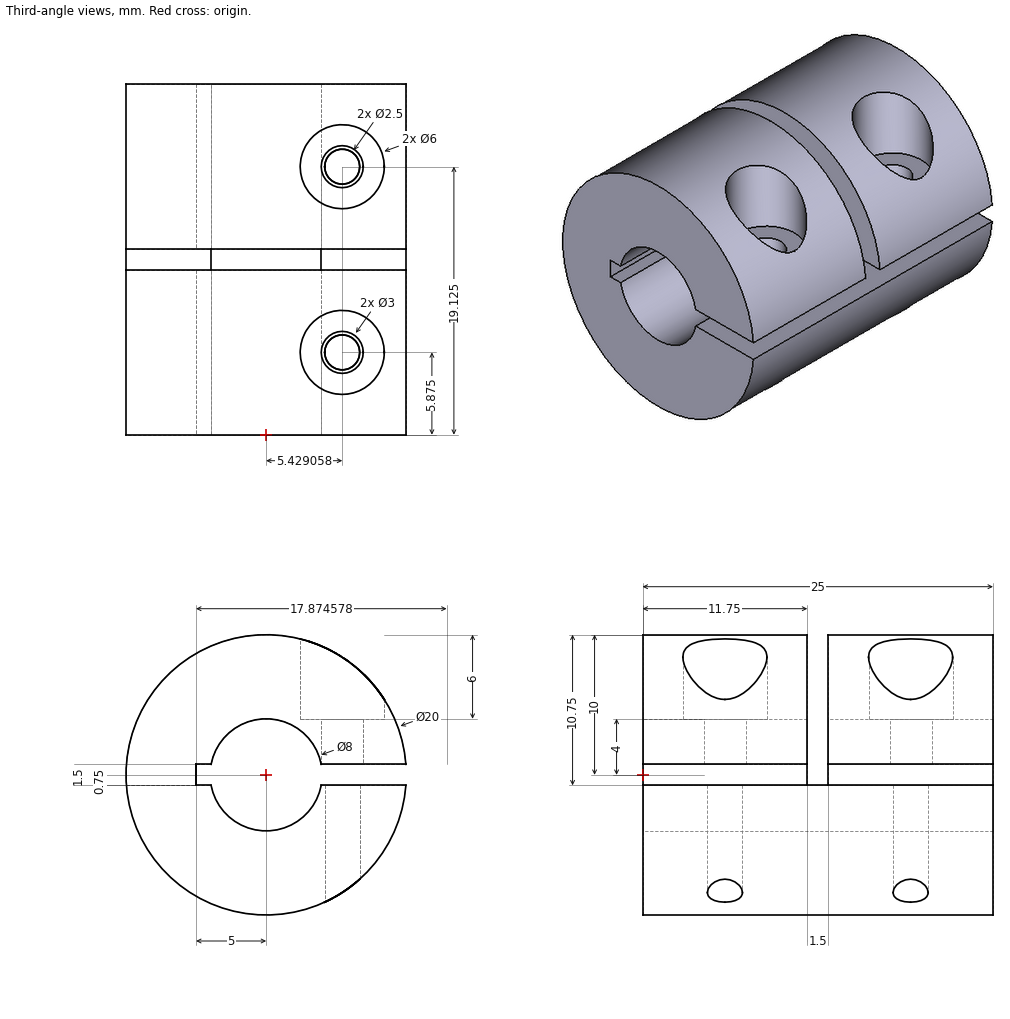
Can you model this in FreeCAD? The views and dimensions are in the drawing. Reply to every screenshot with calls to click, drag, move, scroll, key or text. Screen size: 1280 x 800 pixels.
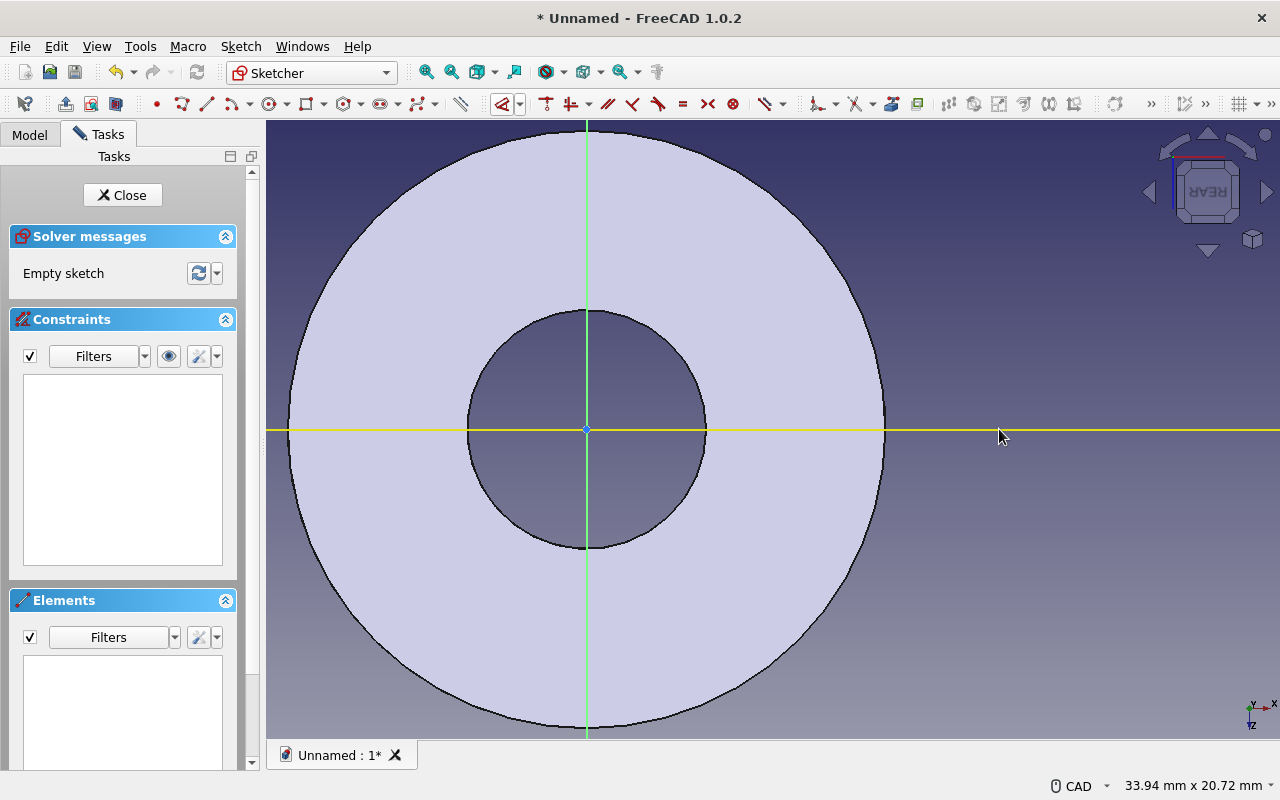
click(306, 104)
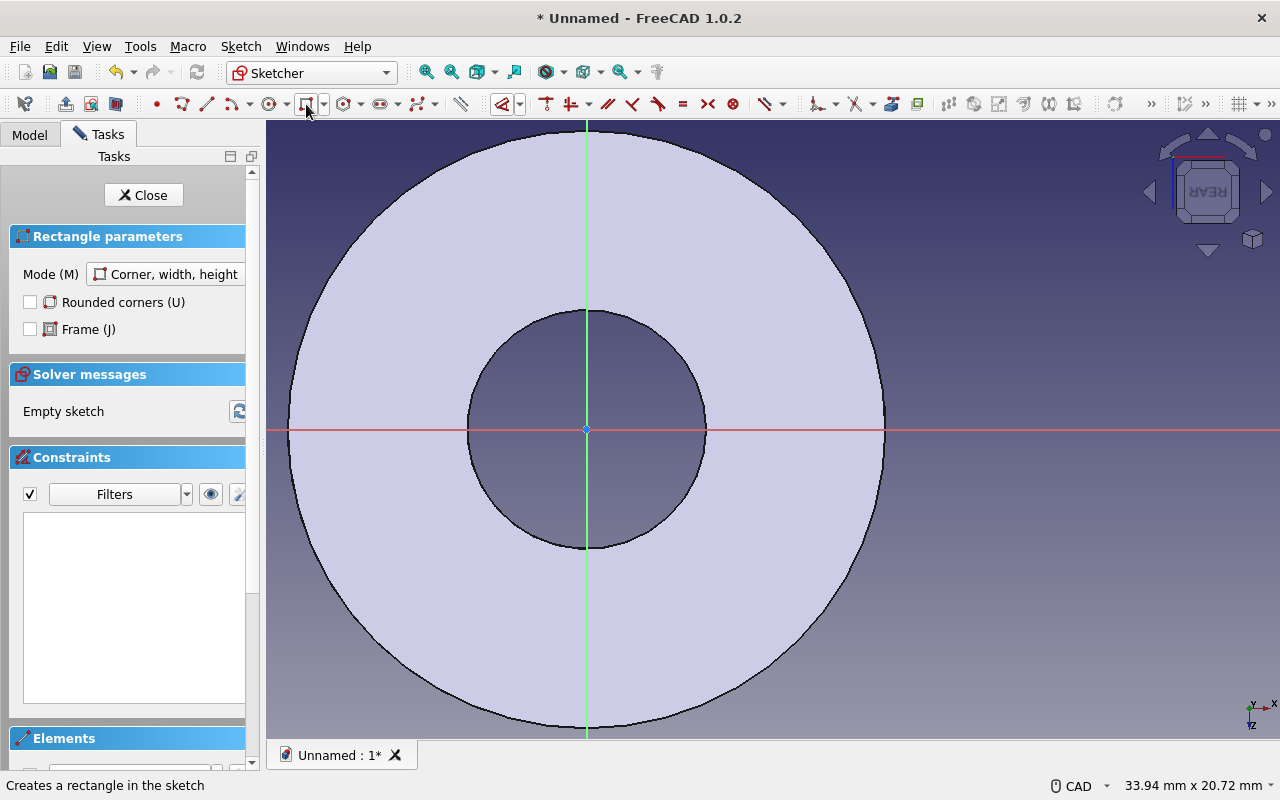
click(437, 407)
click(971, 452)
key(Escape)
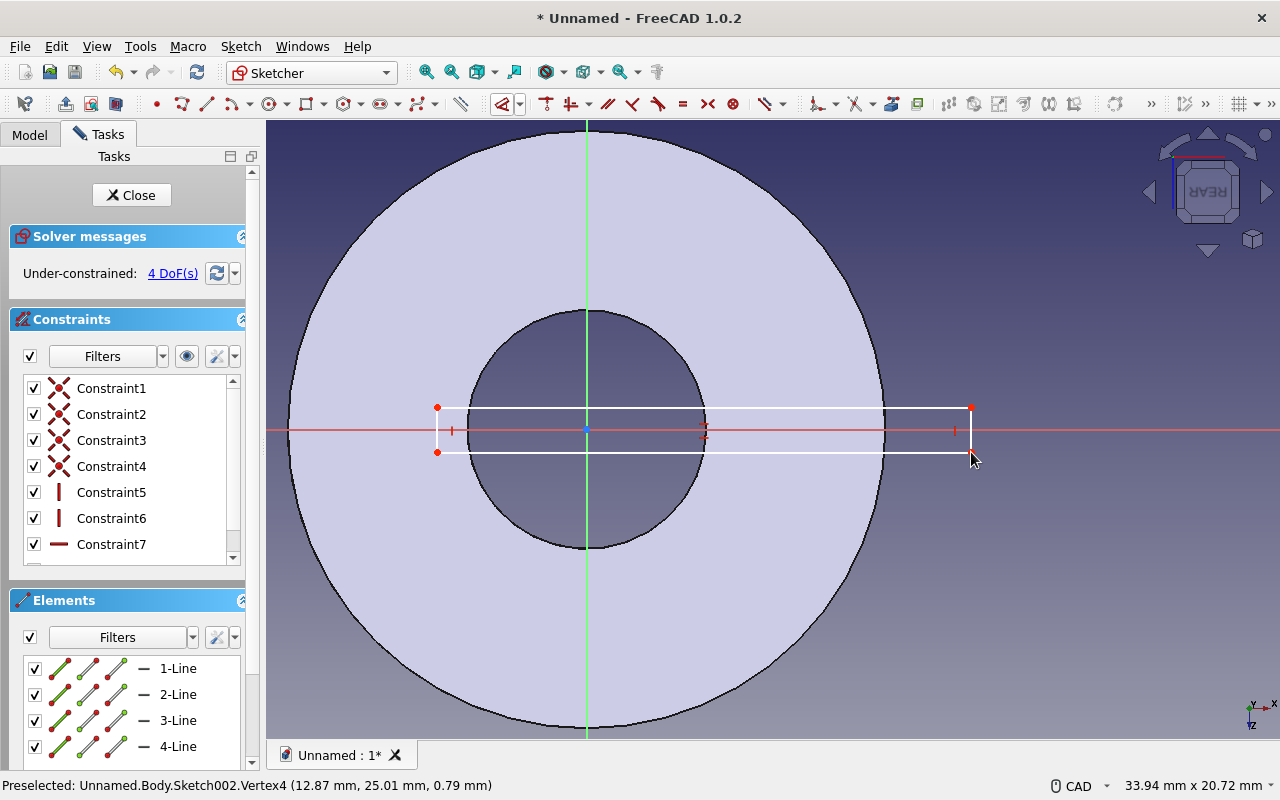
click(437, 408)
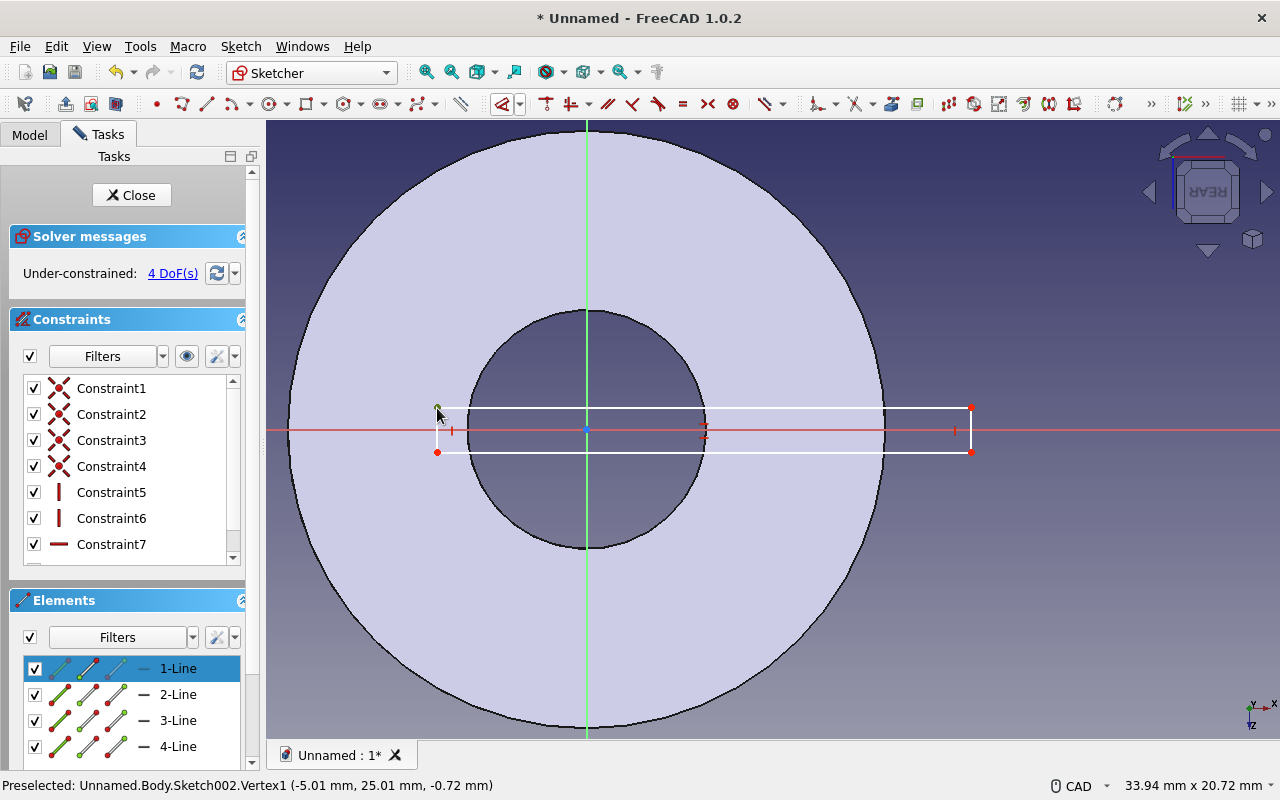
click(520, 104)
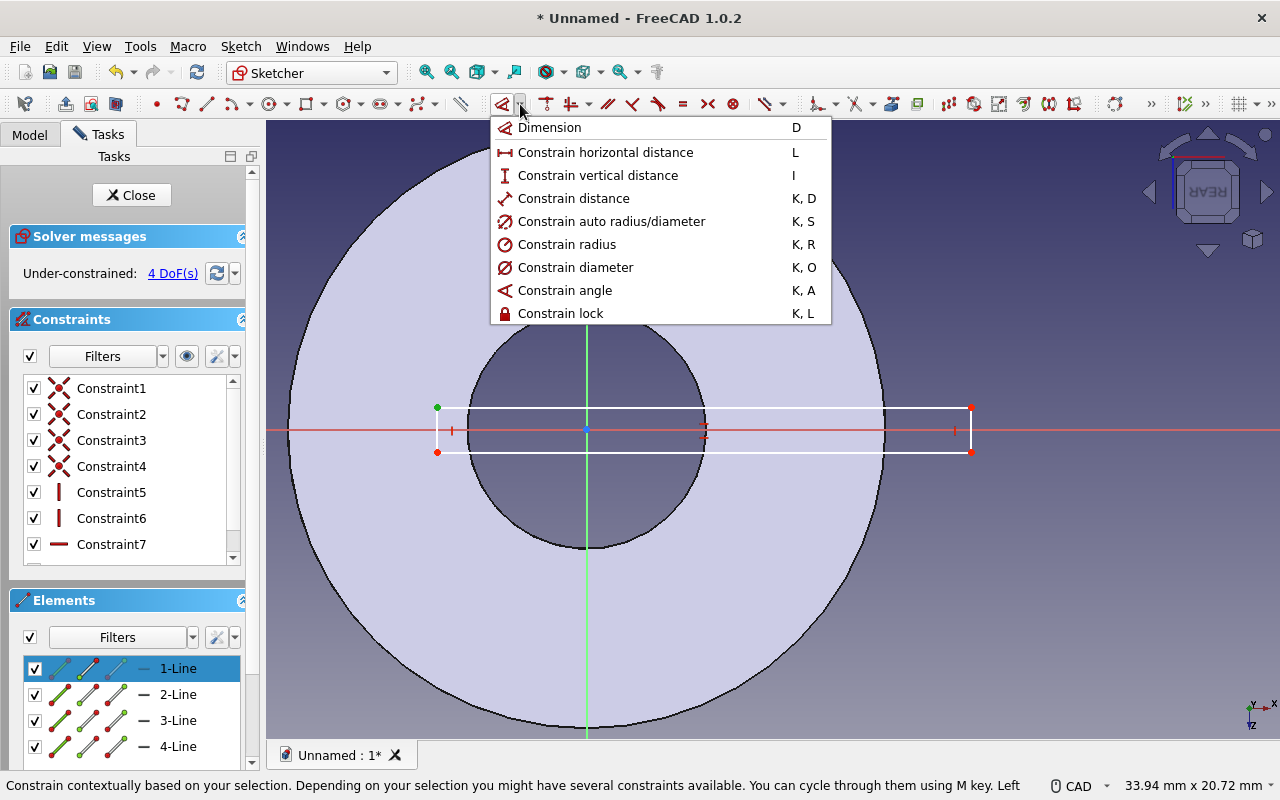
click(661, 152)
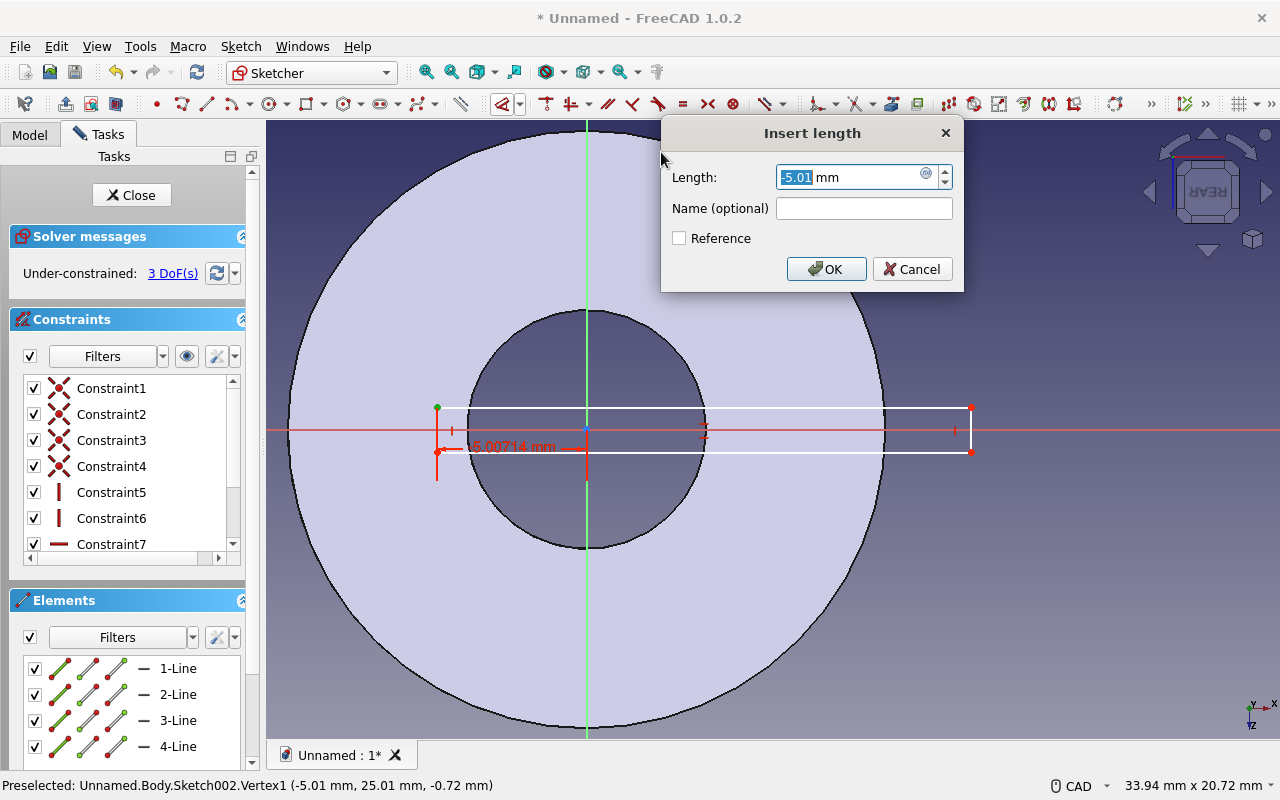
text(-5)
key(Return)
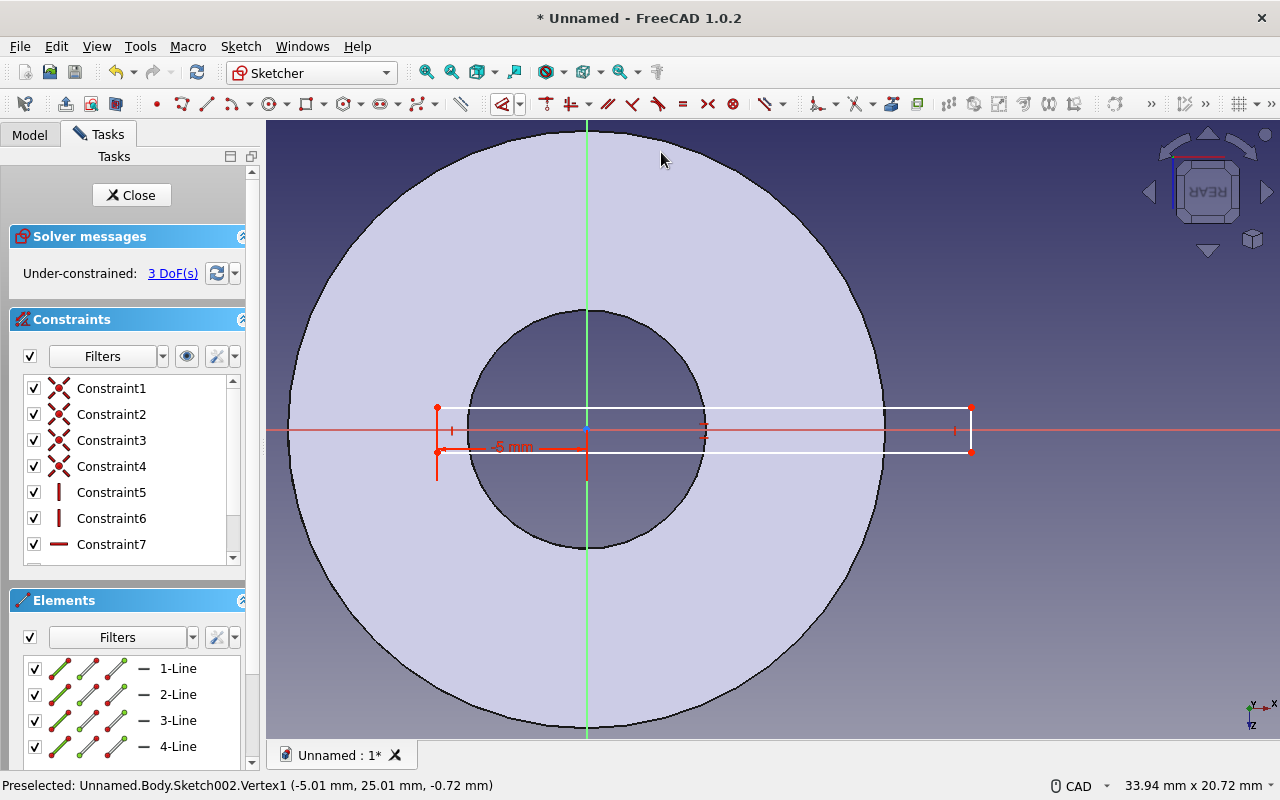
scroll(437, 440, up, 2)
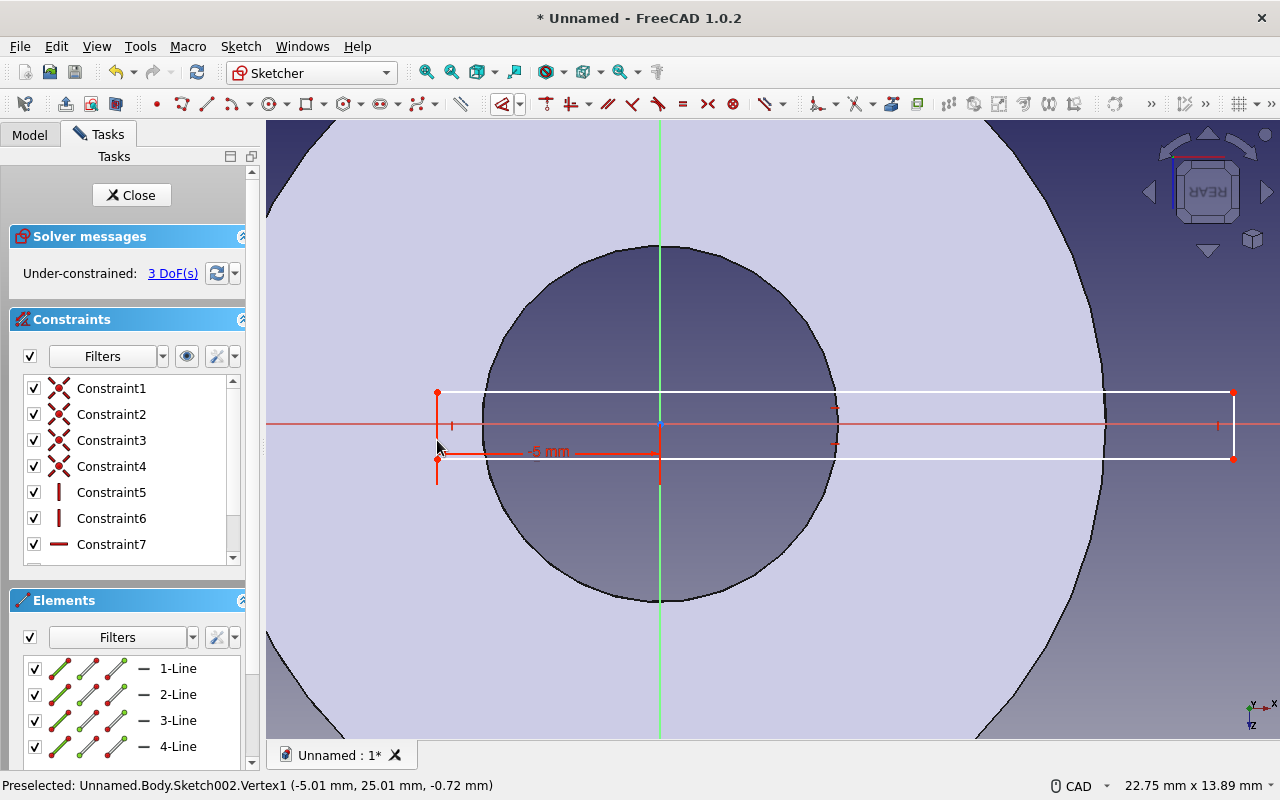
click(437, 439)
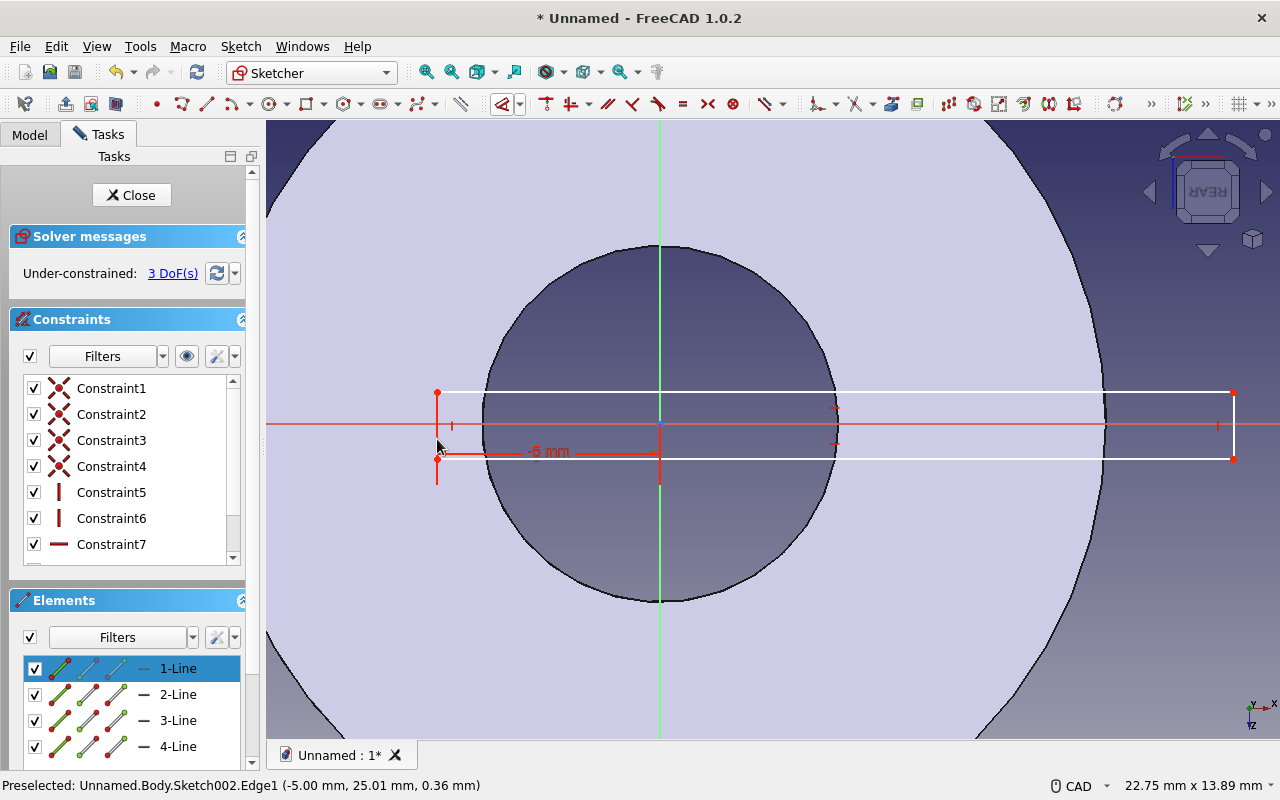
click(520, 104)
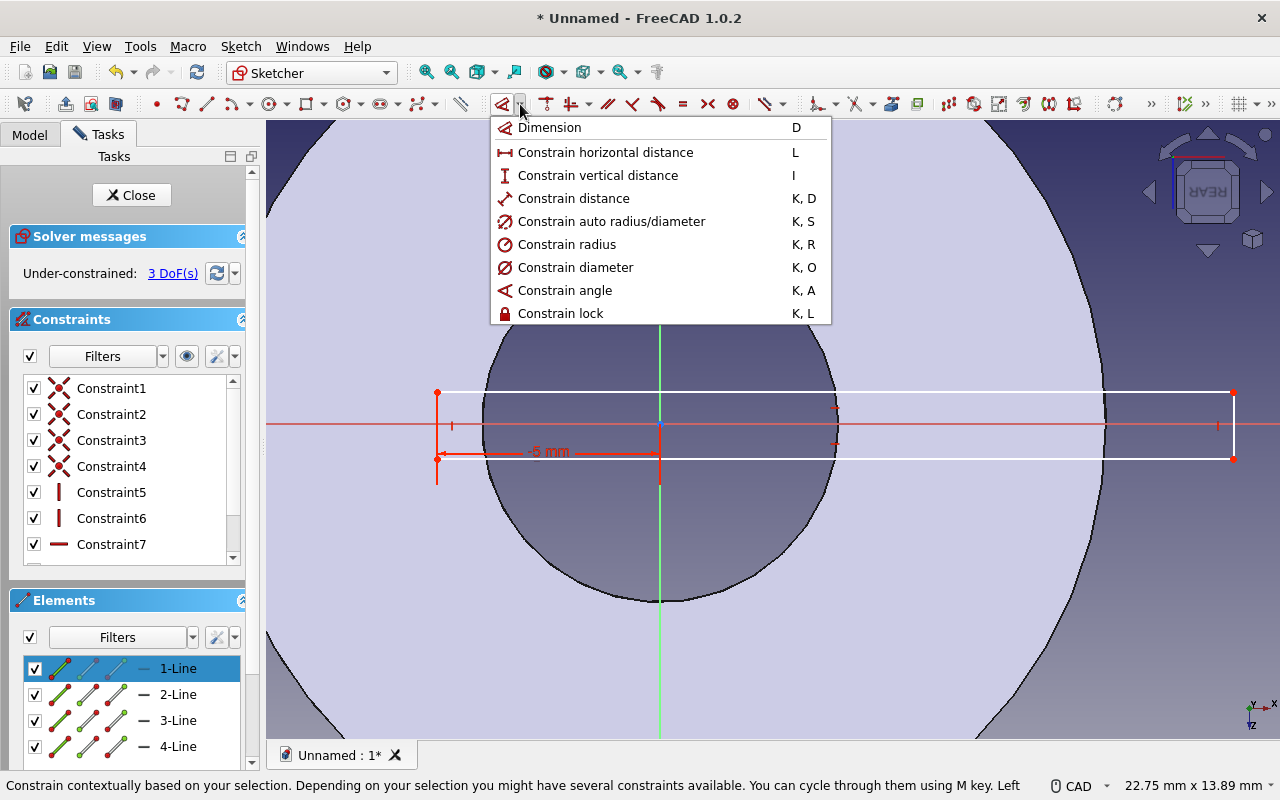
click(661, 176)